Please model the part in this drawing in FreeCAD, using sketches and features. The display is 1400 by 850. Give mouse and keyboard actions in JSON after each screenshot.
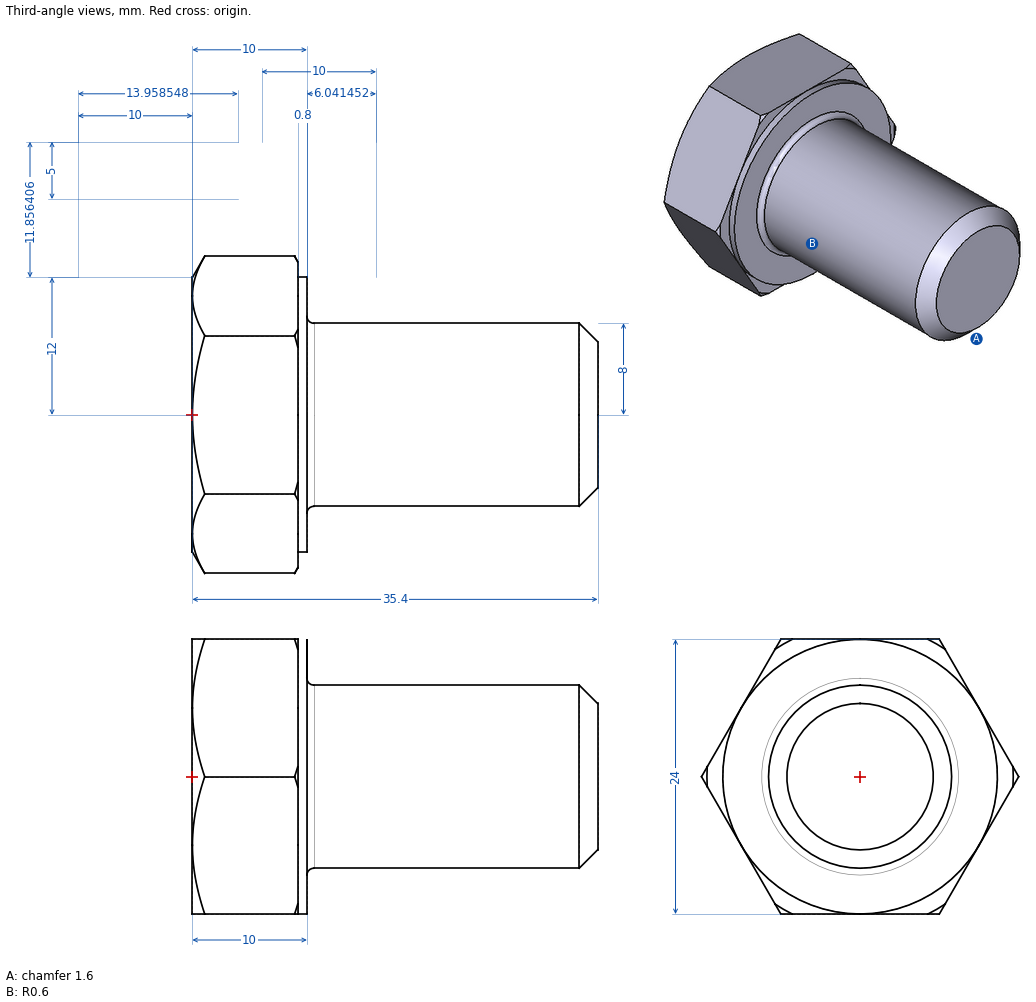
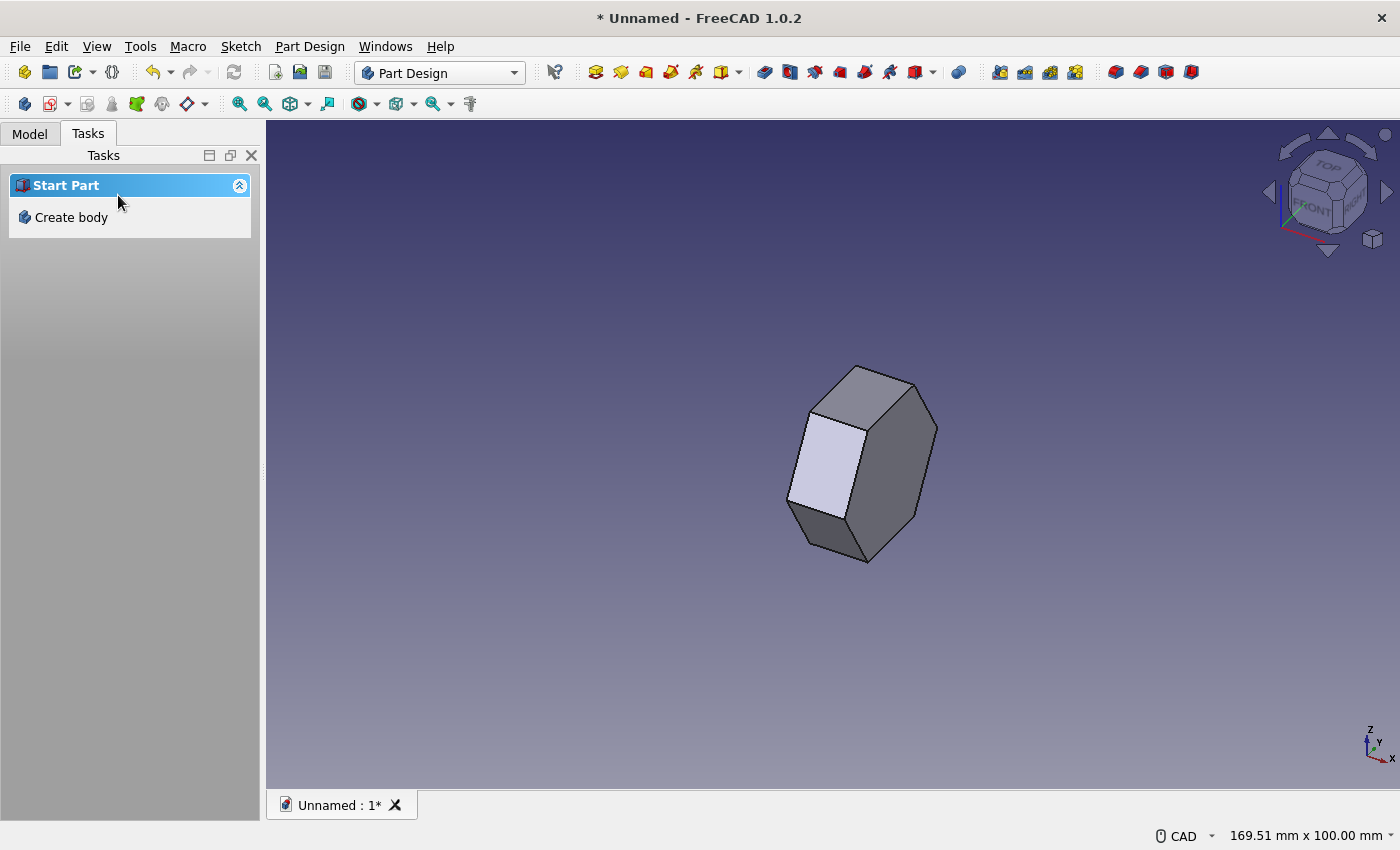
{"action": "left_click", "coordinate": [240, 104]}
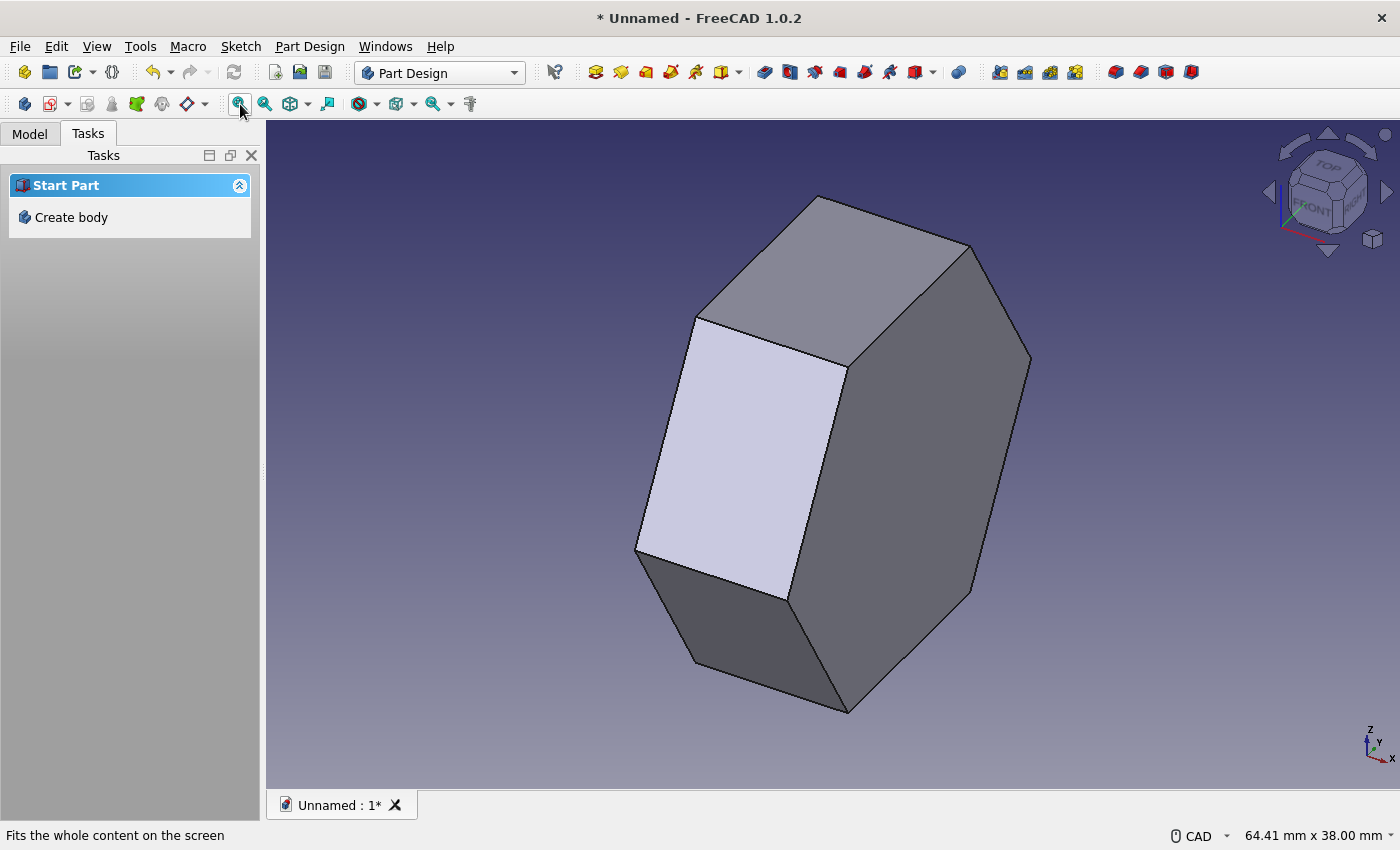
{"action": "left_click", "coordinate": [50, 104]}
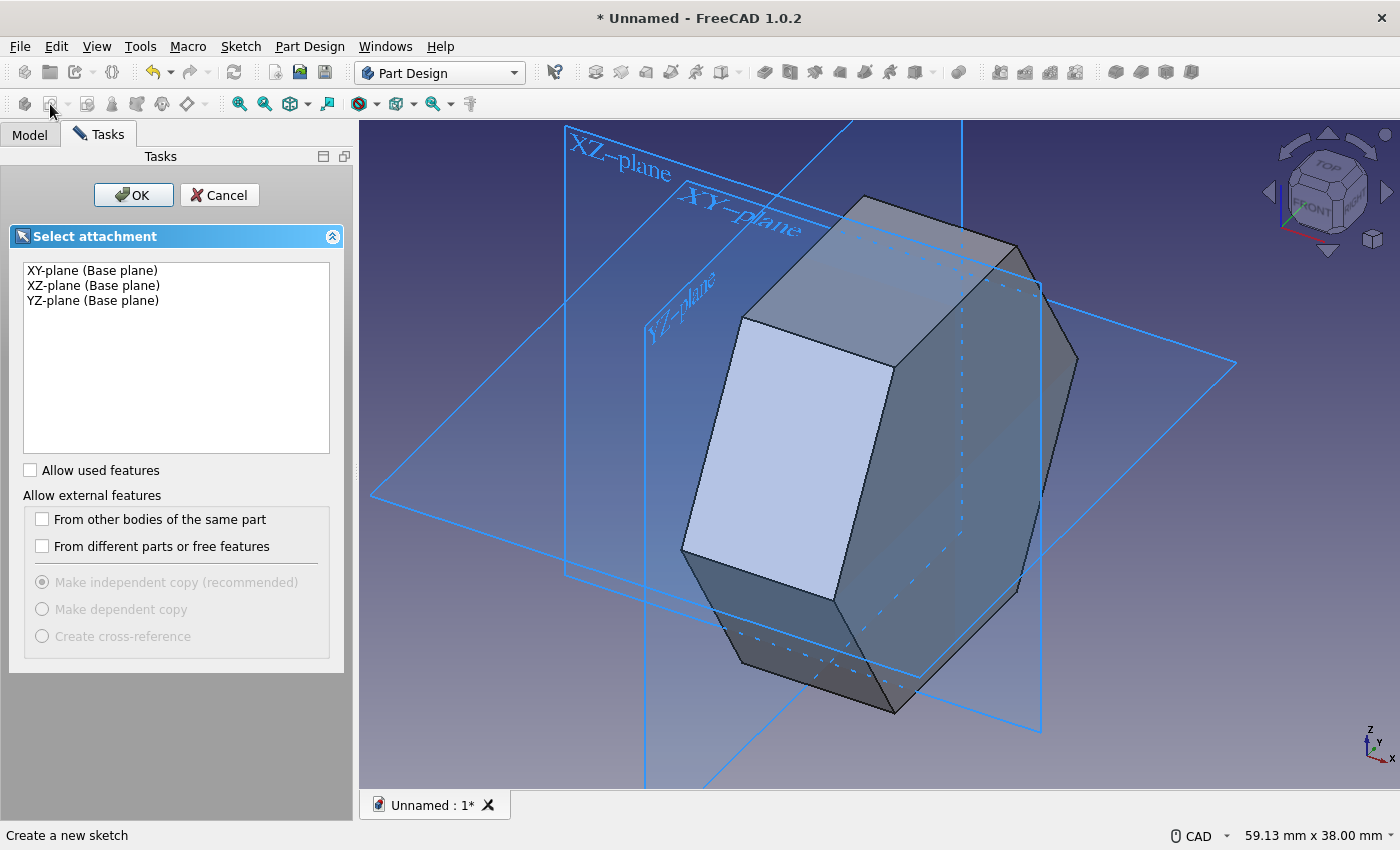
{"action": "left_click", "coordinate": [84, 270]}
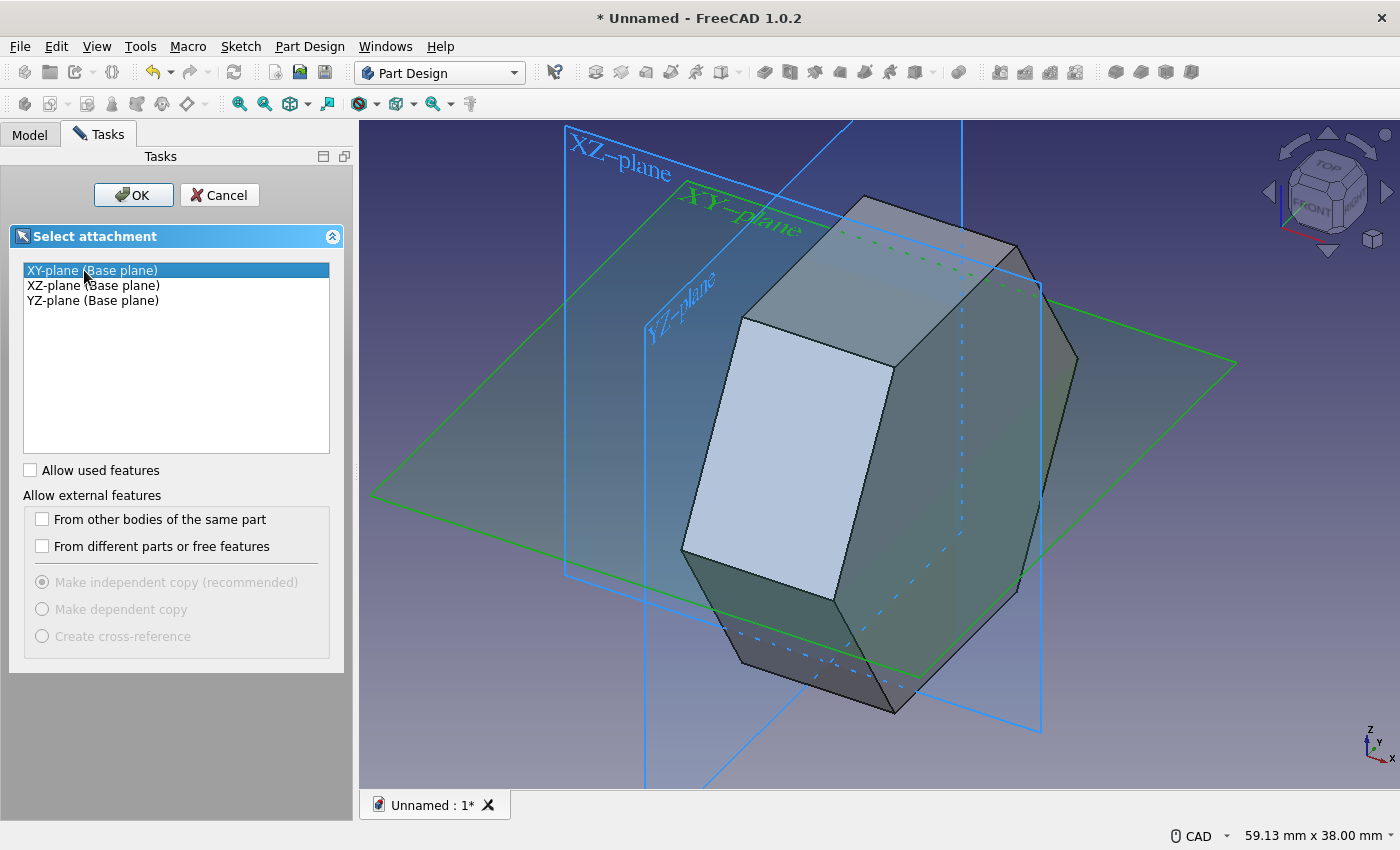
{"action": "left_click", "coordinate": [134, 195]}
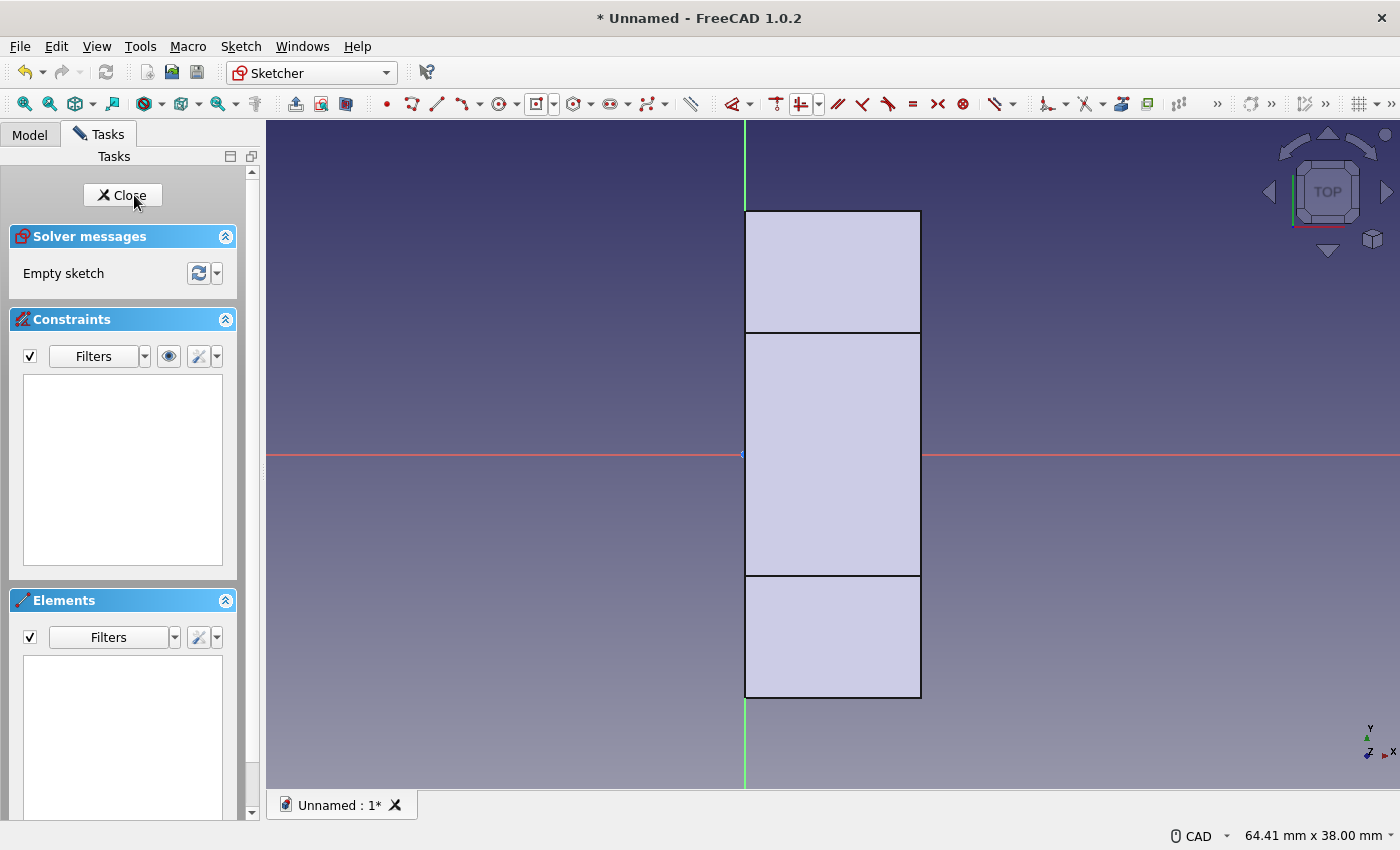
{"action": "left_click", "coordinate": [346, 104]}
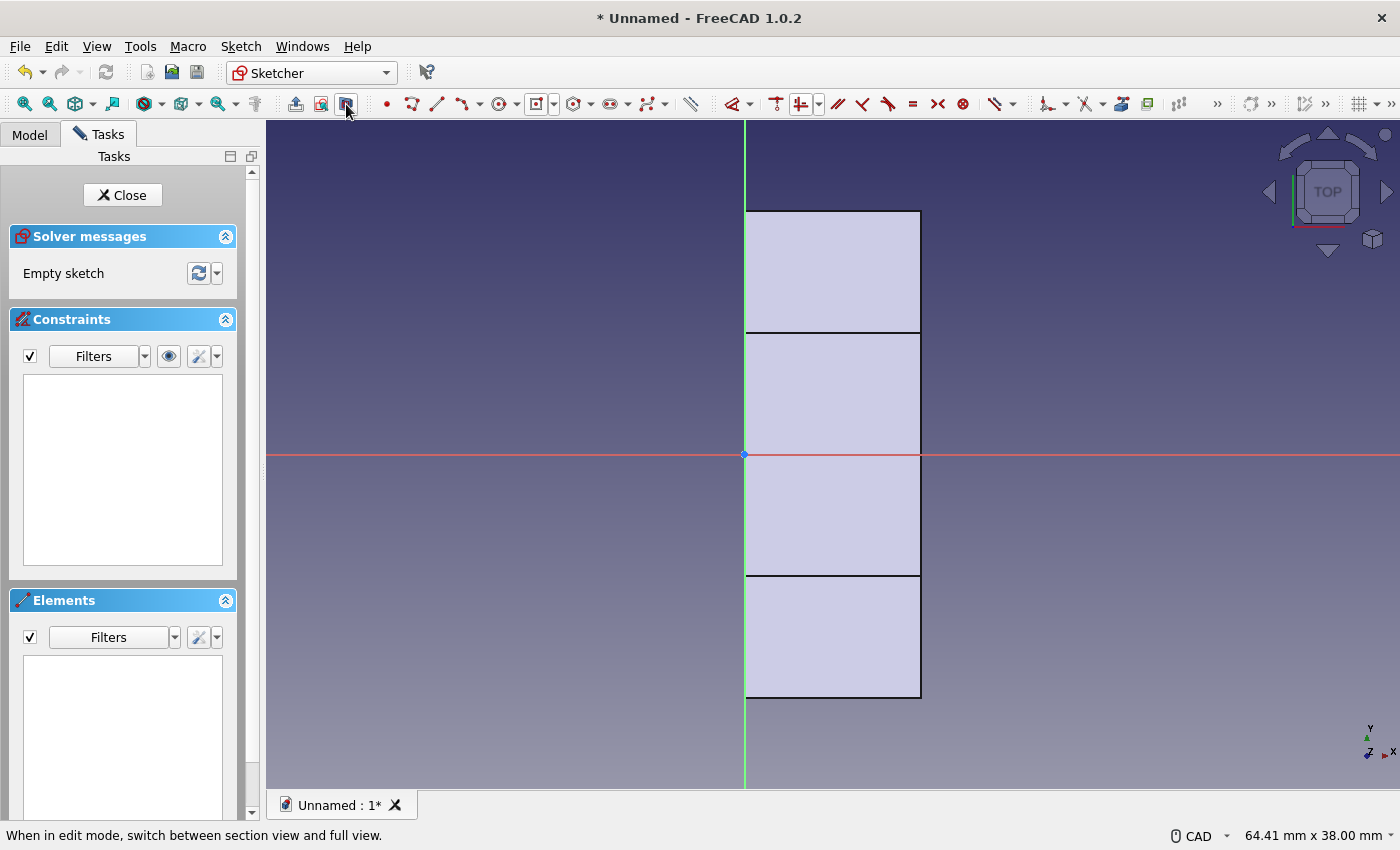
{"action": "scroll", "coordinate": [294, 761], "scroll_direction": "down", "scroll_amount": 1}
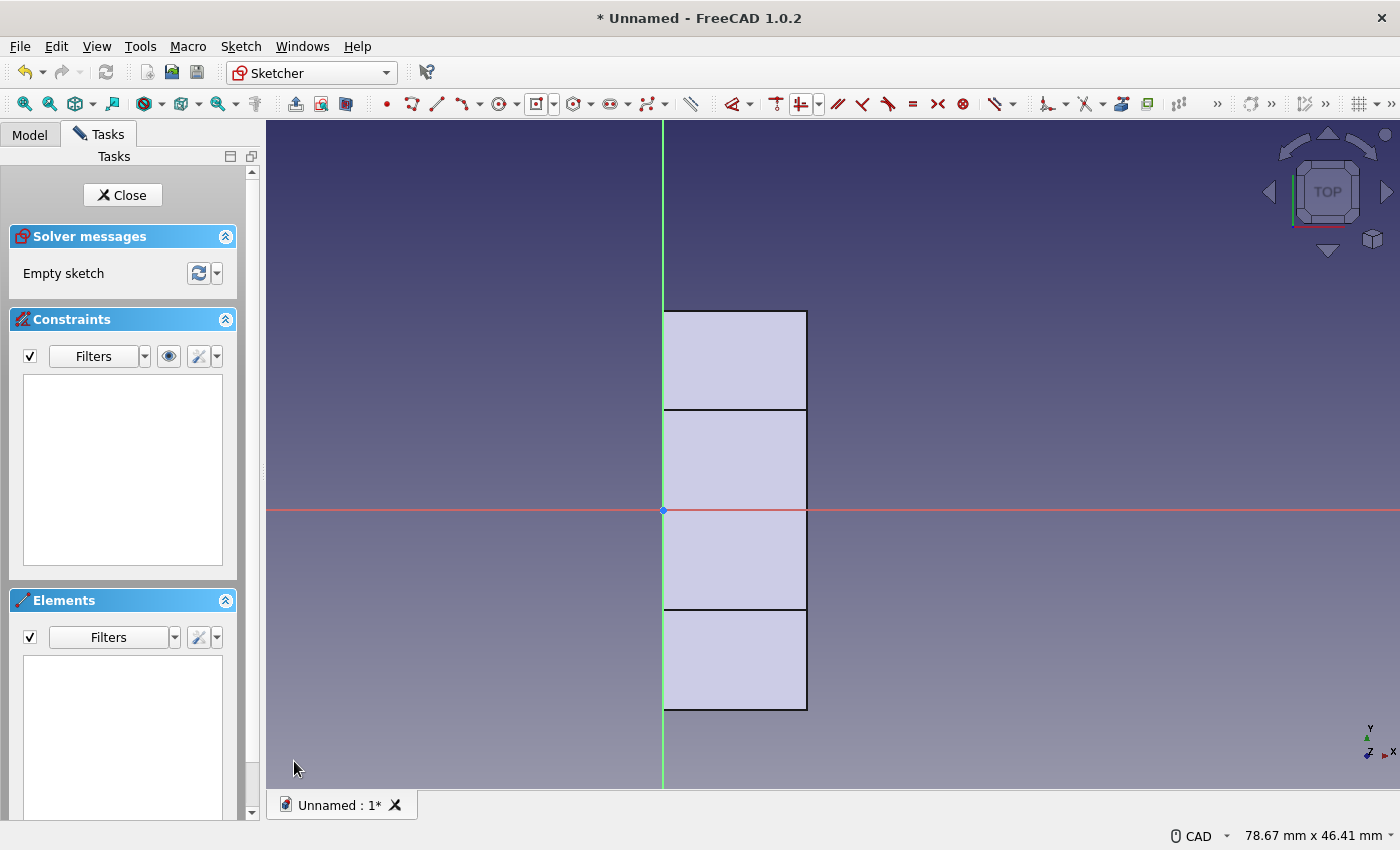
{"action": "key", "text": "g r"}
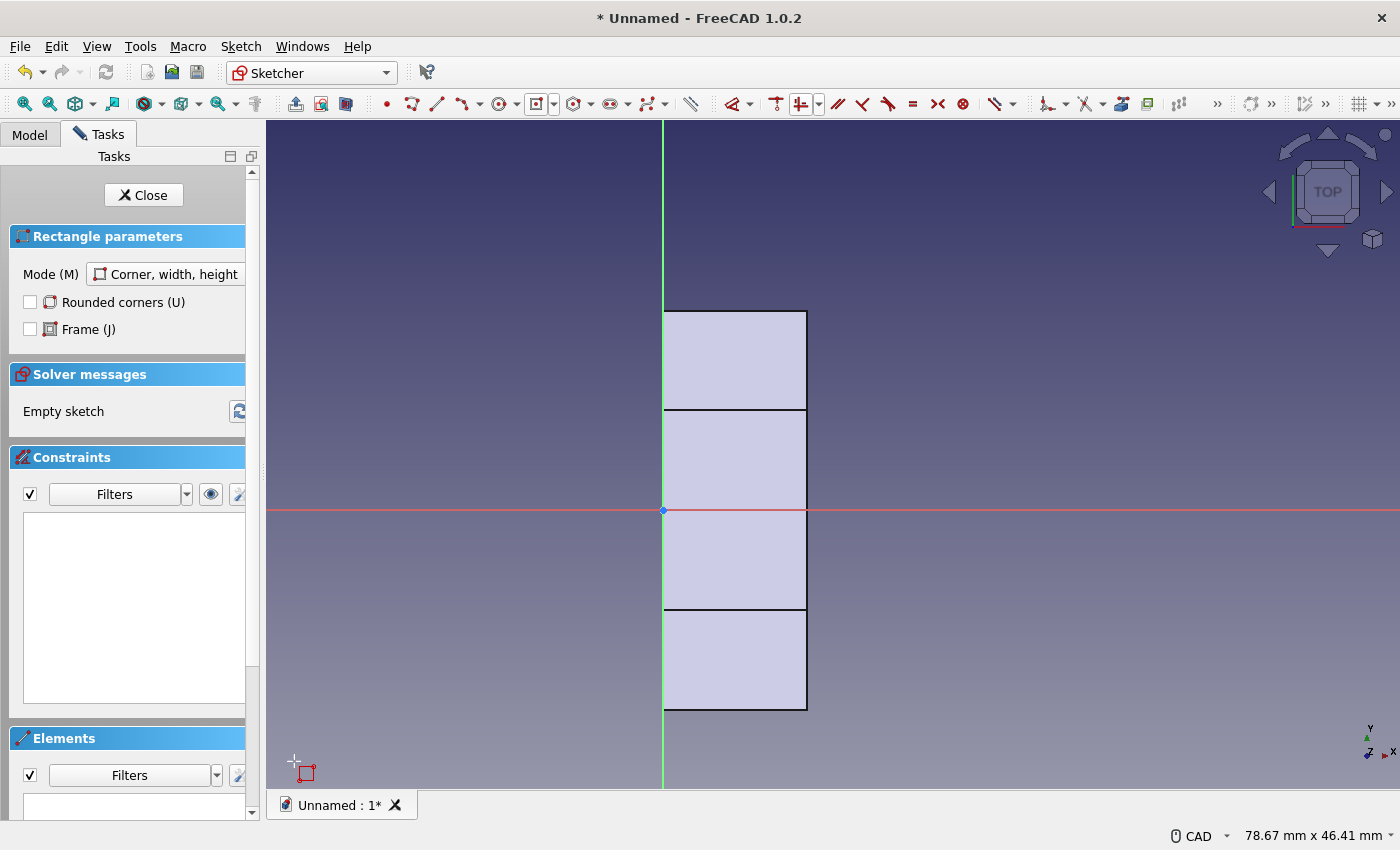
{"action": "left_click", "coordinate": [663, 510]}
{"action": "mouse_move", "coordinate": [1173, 395]}